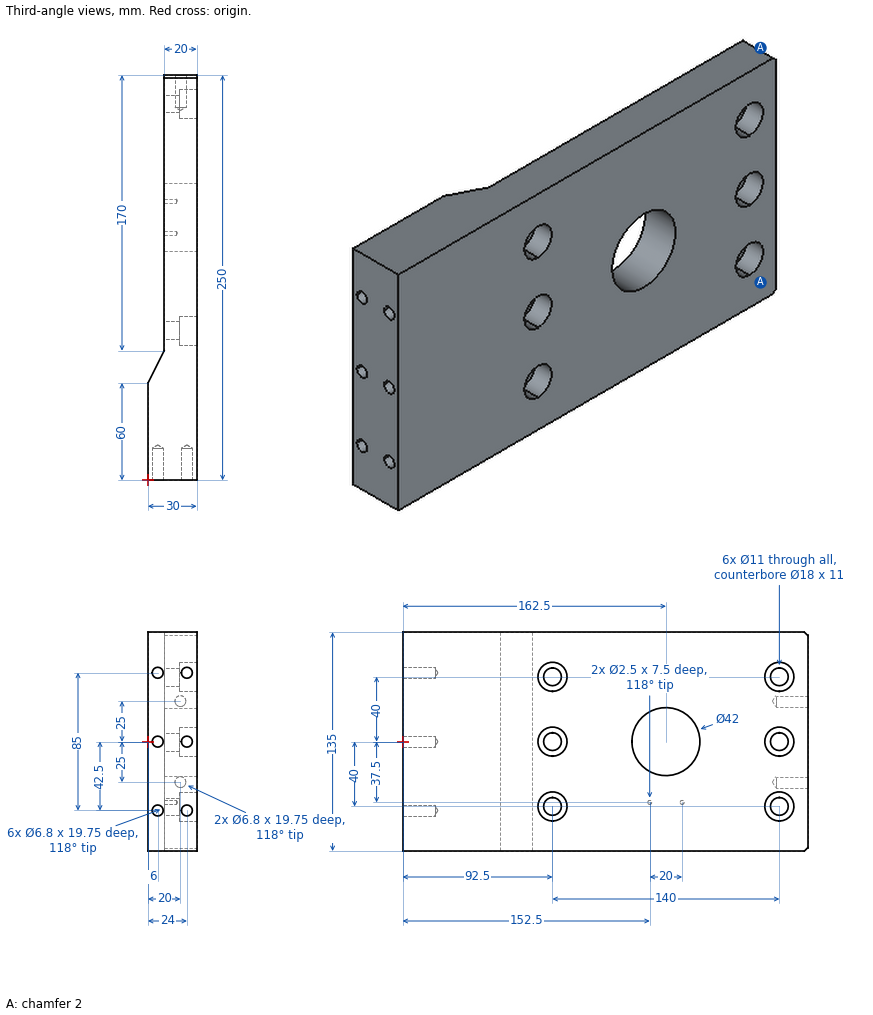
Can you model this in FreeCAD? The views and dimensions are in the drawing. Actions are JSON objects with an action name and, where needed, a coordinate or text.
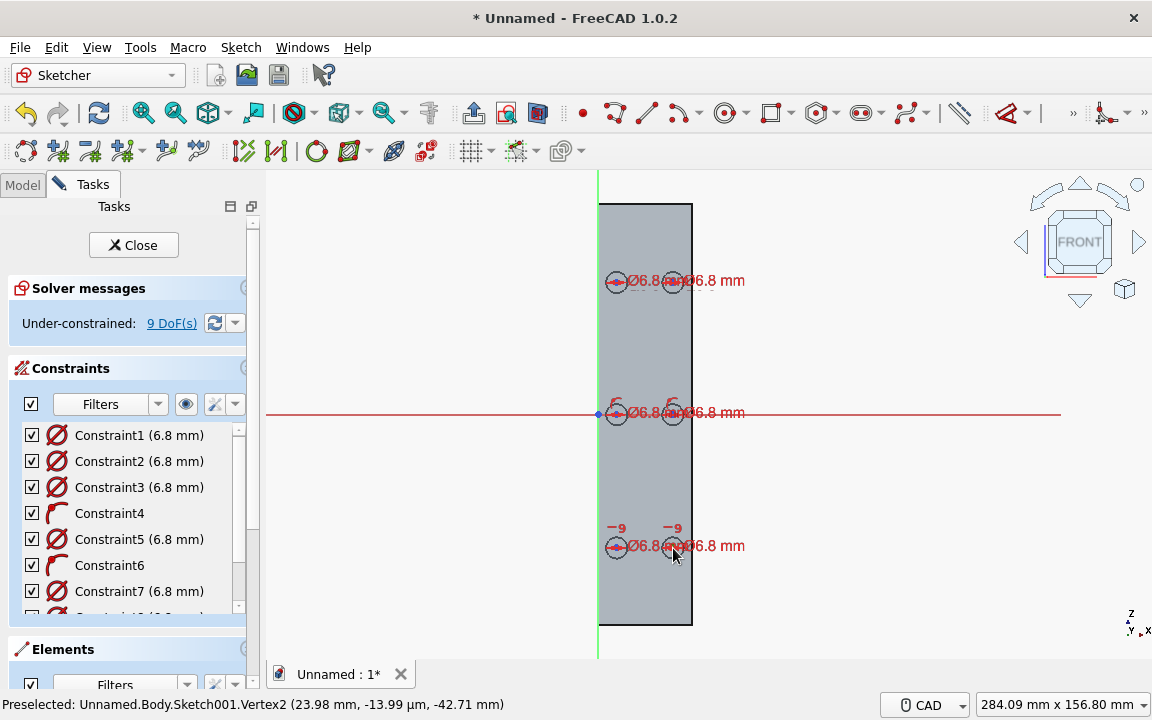
{"action": "left_click", "coordinate": [673, 415]}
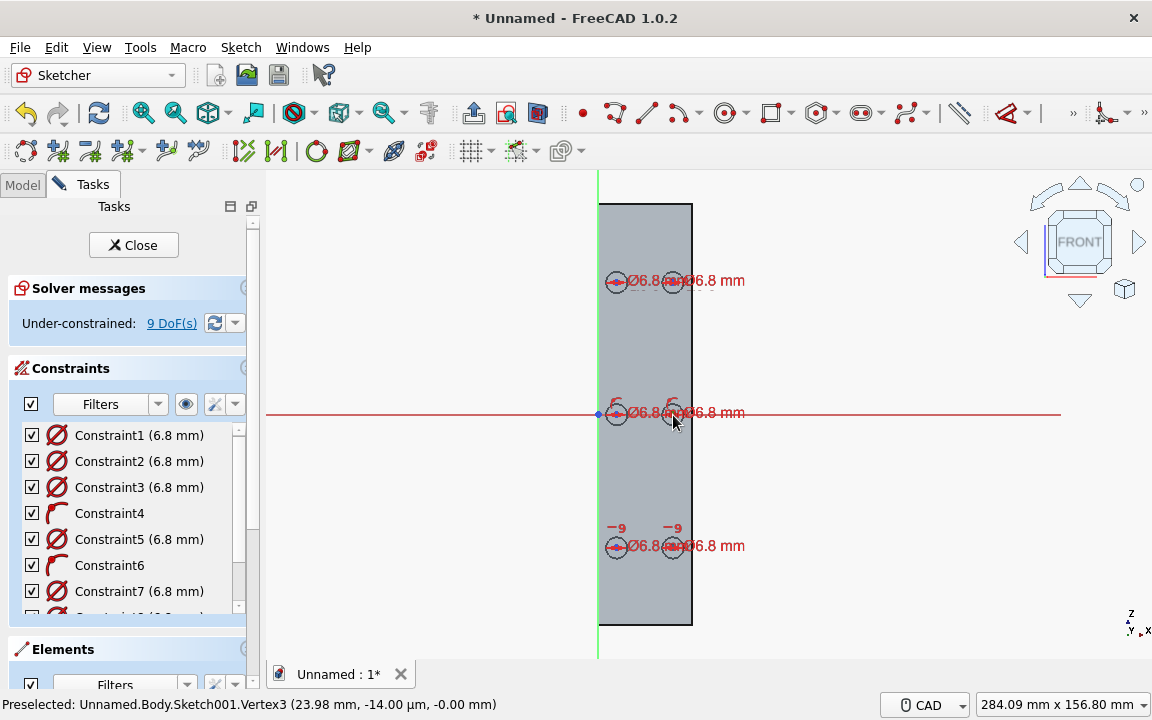
{"action": "key", "text": "v"}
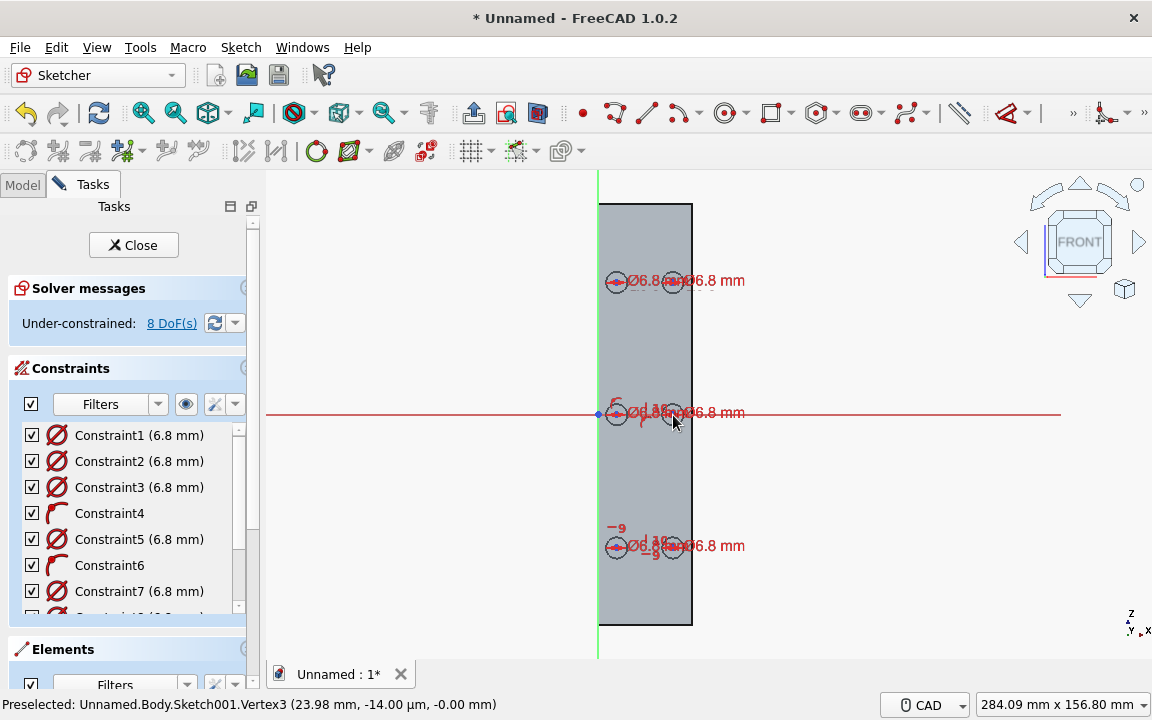
{"action": "left_click", "coordinate": [617, 548]}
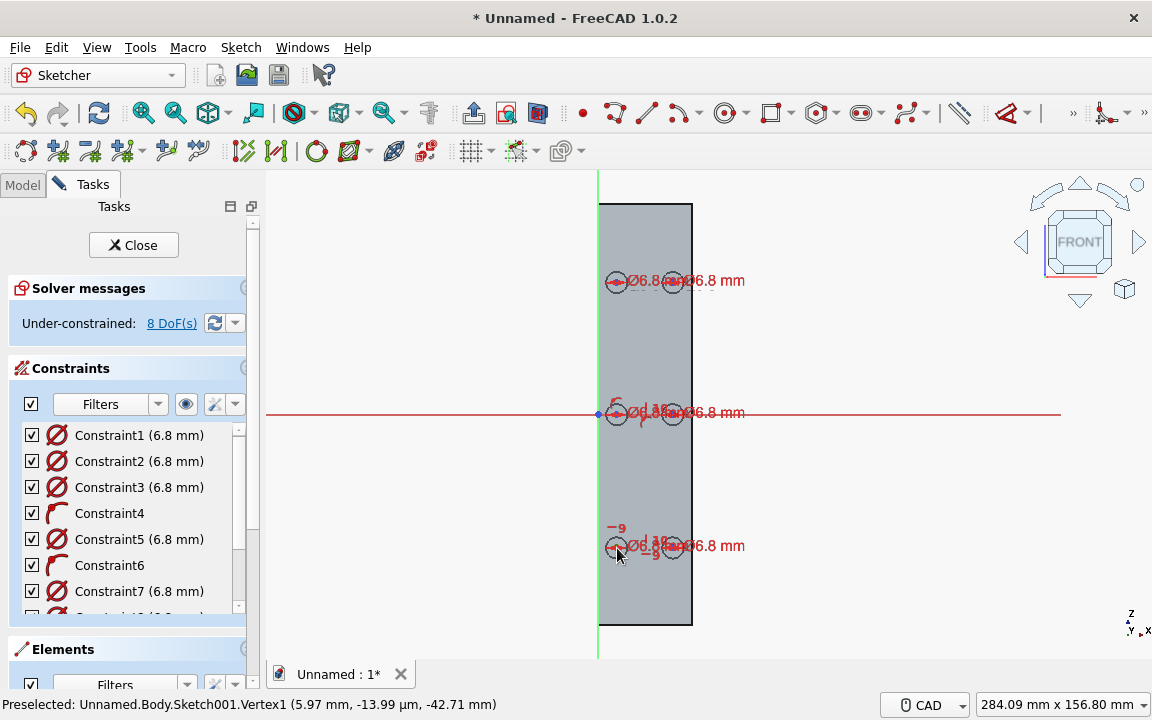
{"action": "left_click", "coordinate": [617, 415]}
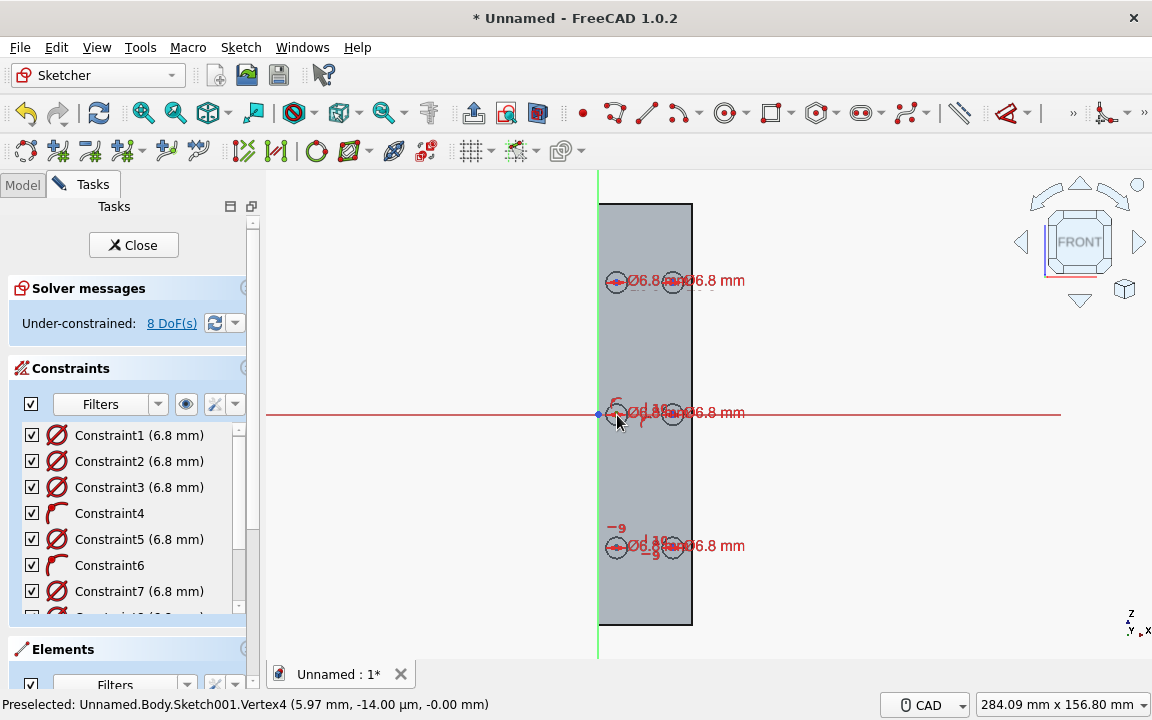
{"action": "key", "text": "v"}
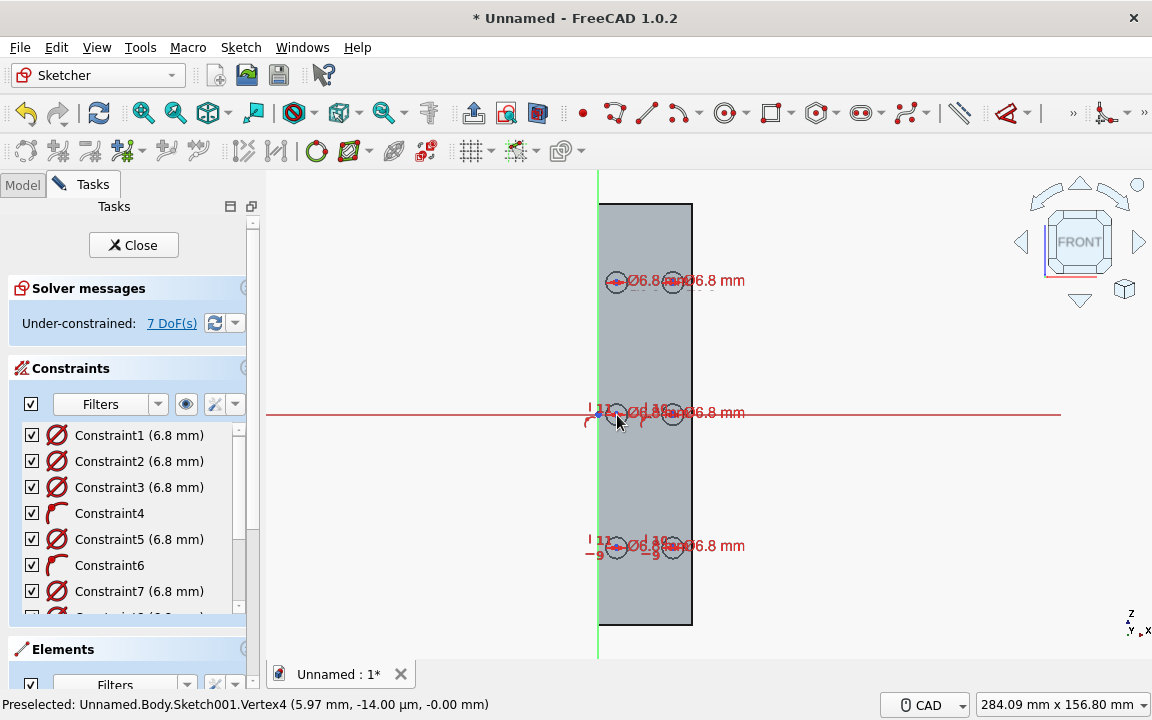
{"action": "left_click", "coordinate": [617, 415]}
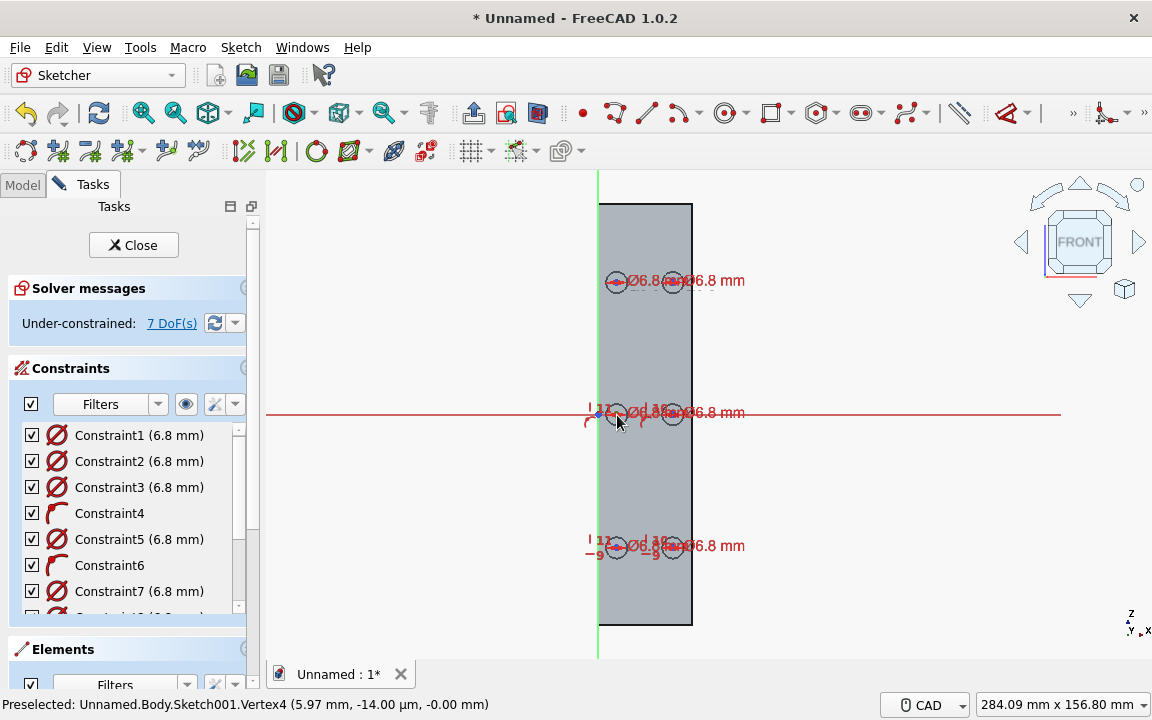
{"action": "left_click", "coordinate": [617, 283]}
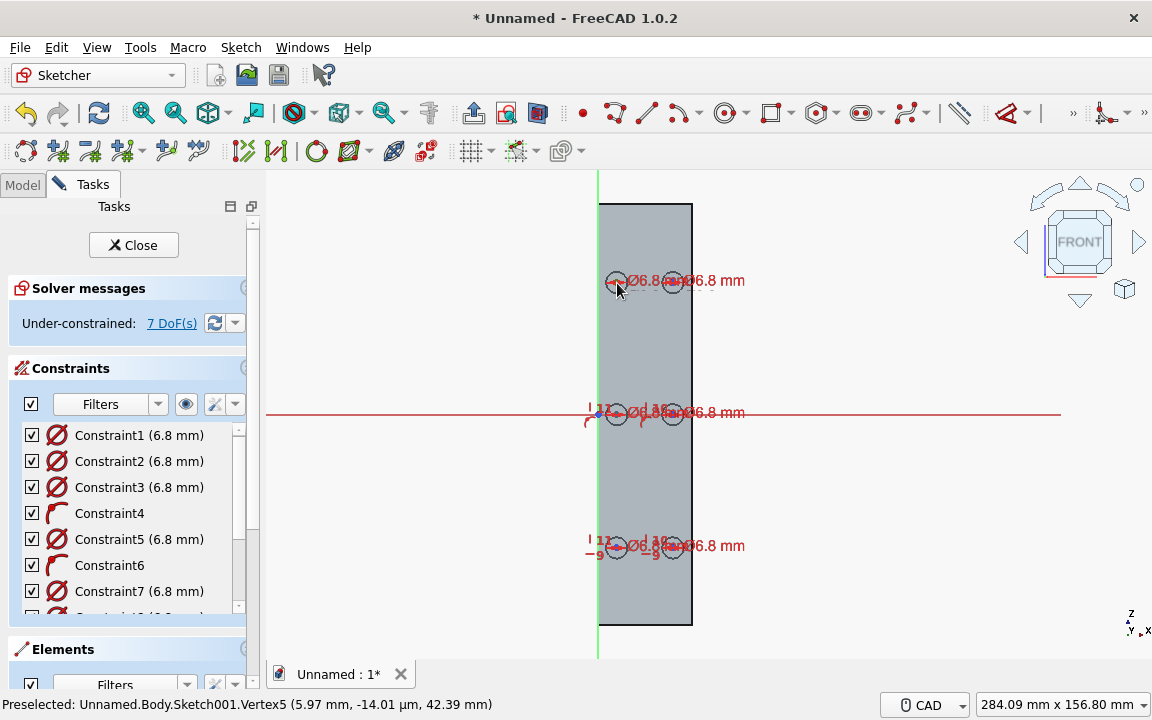
{"action": "key", "text": "v"}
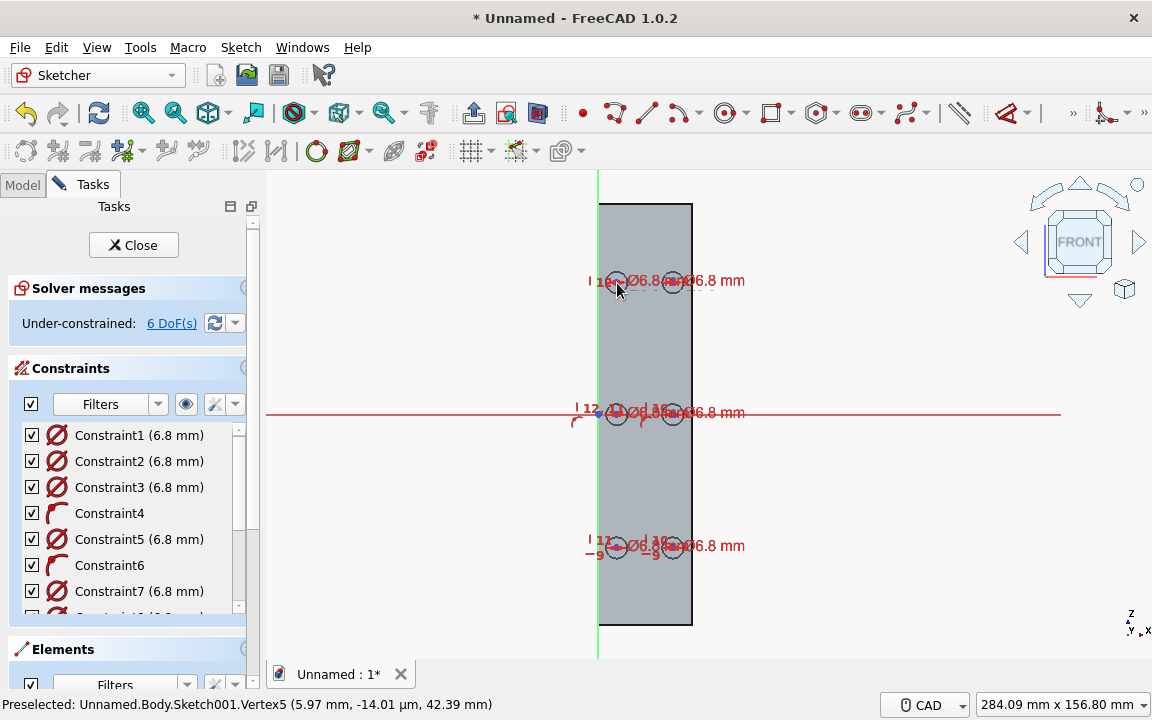
{"action": "left_click", "coordinate": [673, 415]}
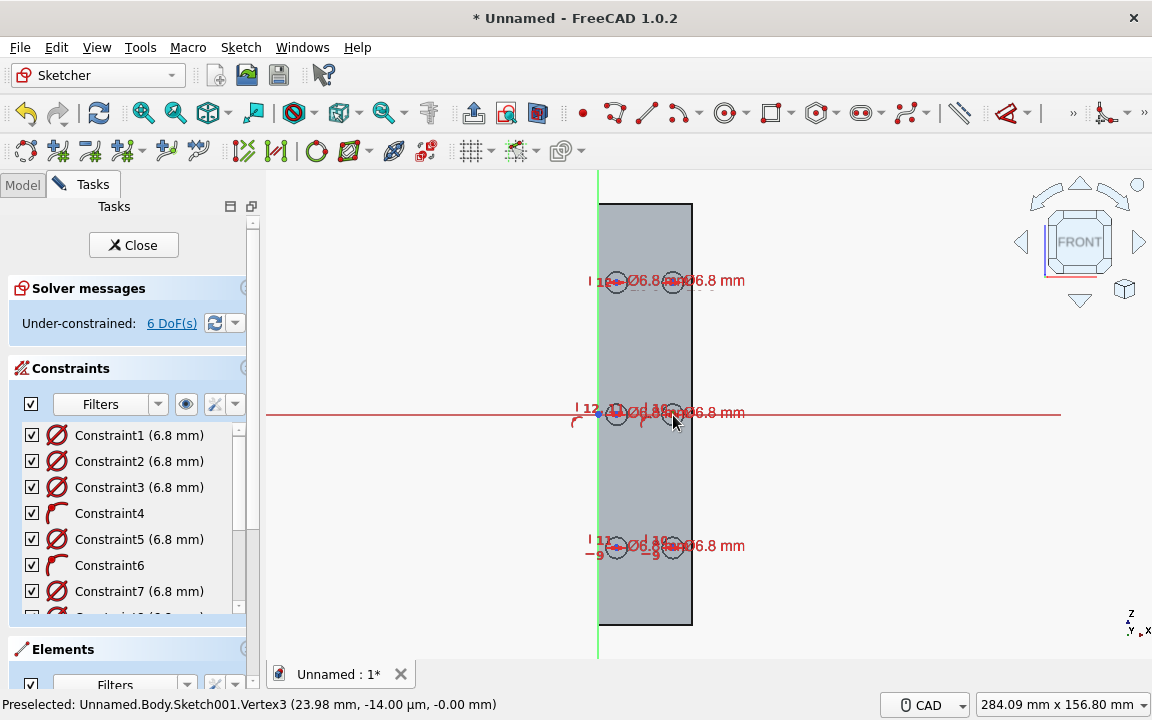
{"action": "left_click", "coordinate": [673, 283]}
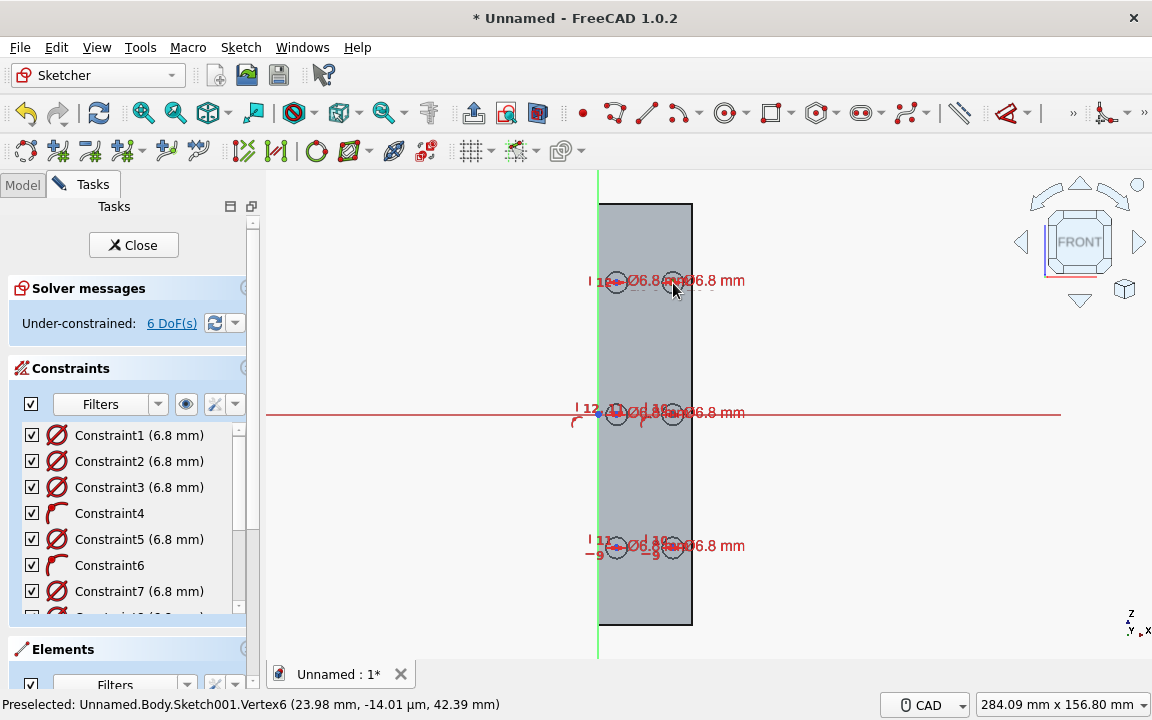
{"action": "key", "text": "v"}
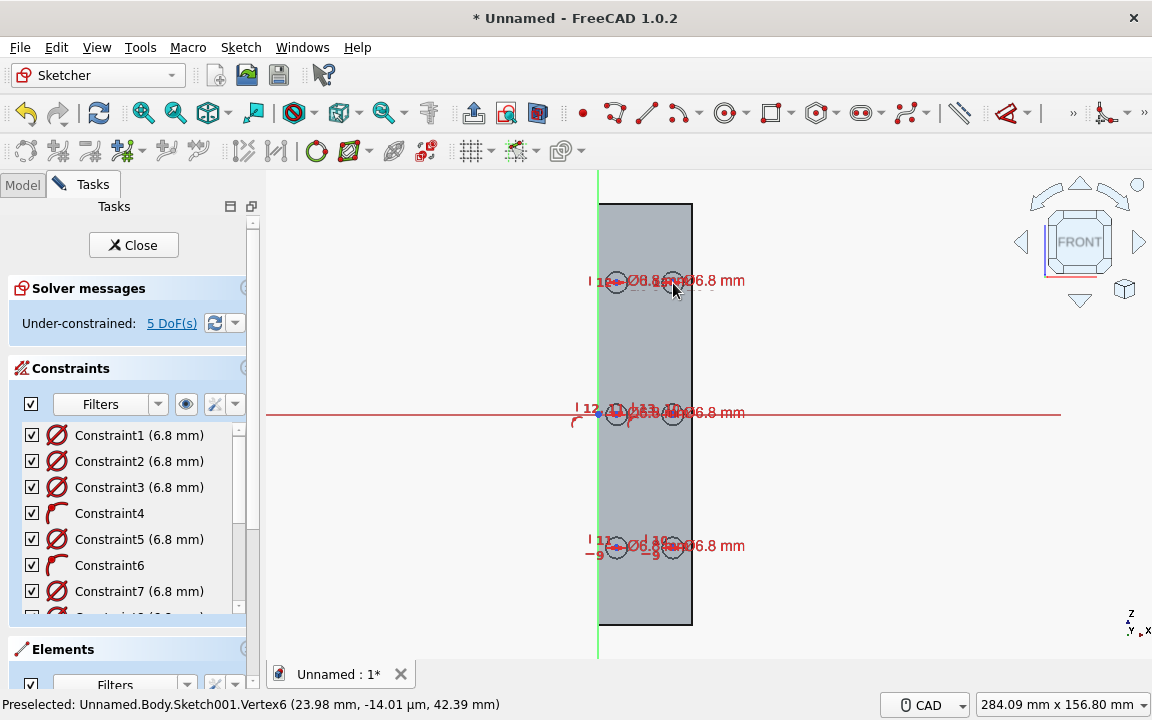
{"action": "left_click", "coordinate": [617, 283]}